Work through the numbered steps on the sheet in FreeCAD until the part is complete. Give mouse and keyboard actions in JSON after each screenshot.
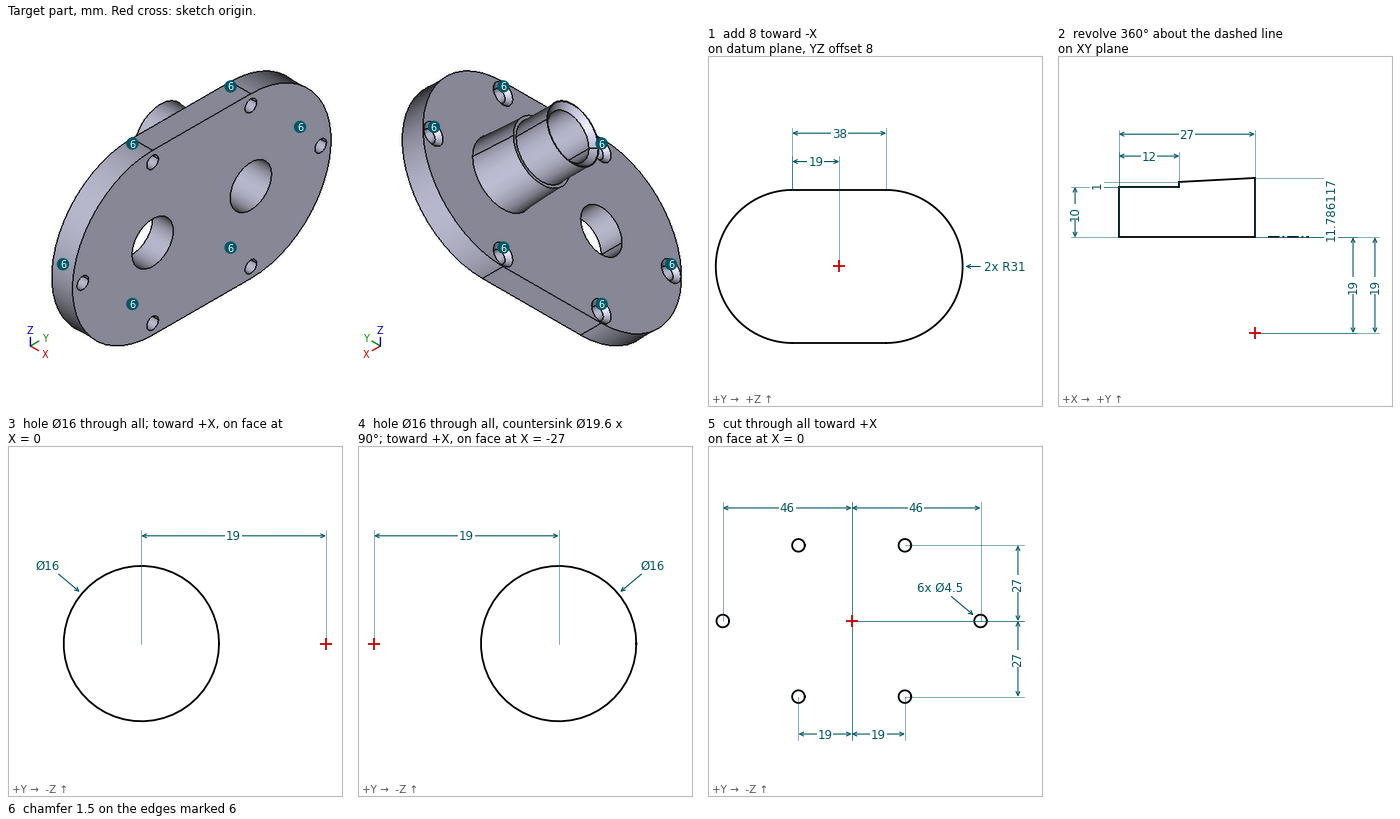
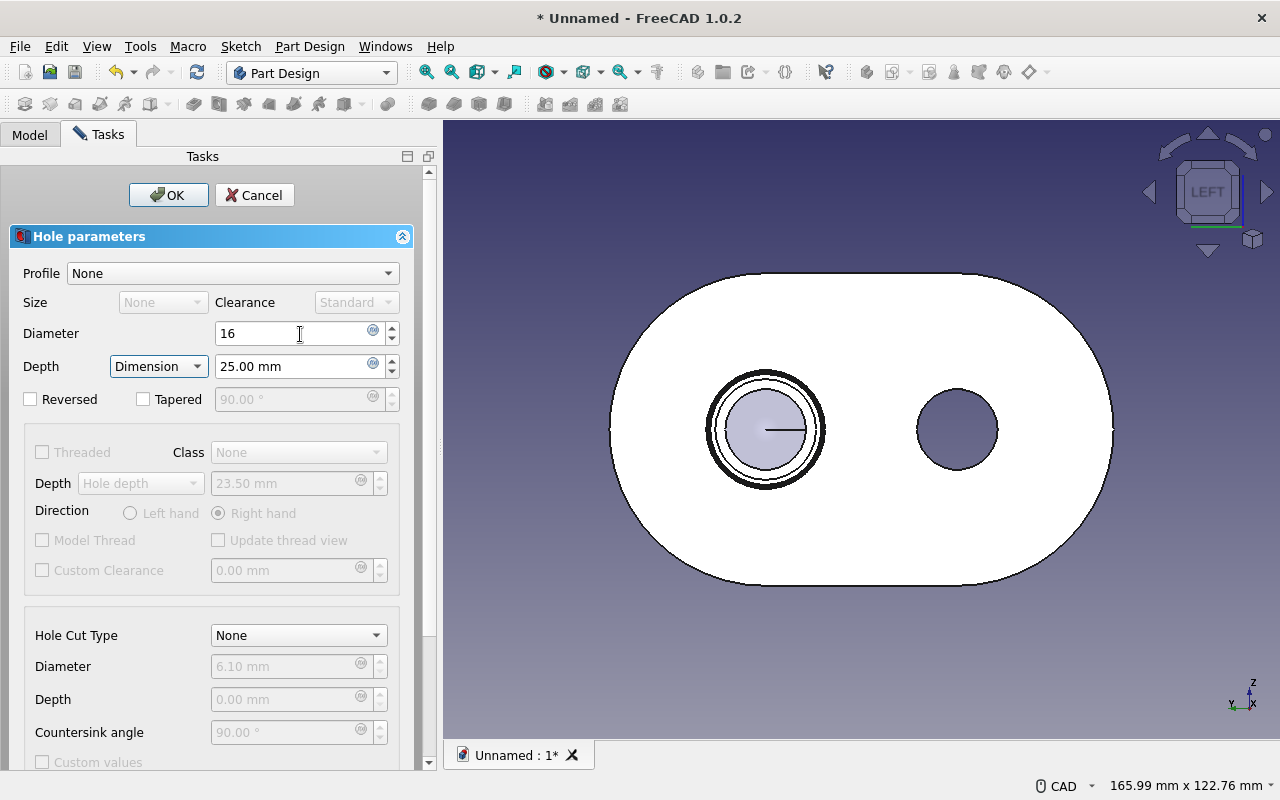
{"action": "left_click", "coordinate": [160, 366]}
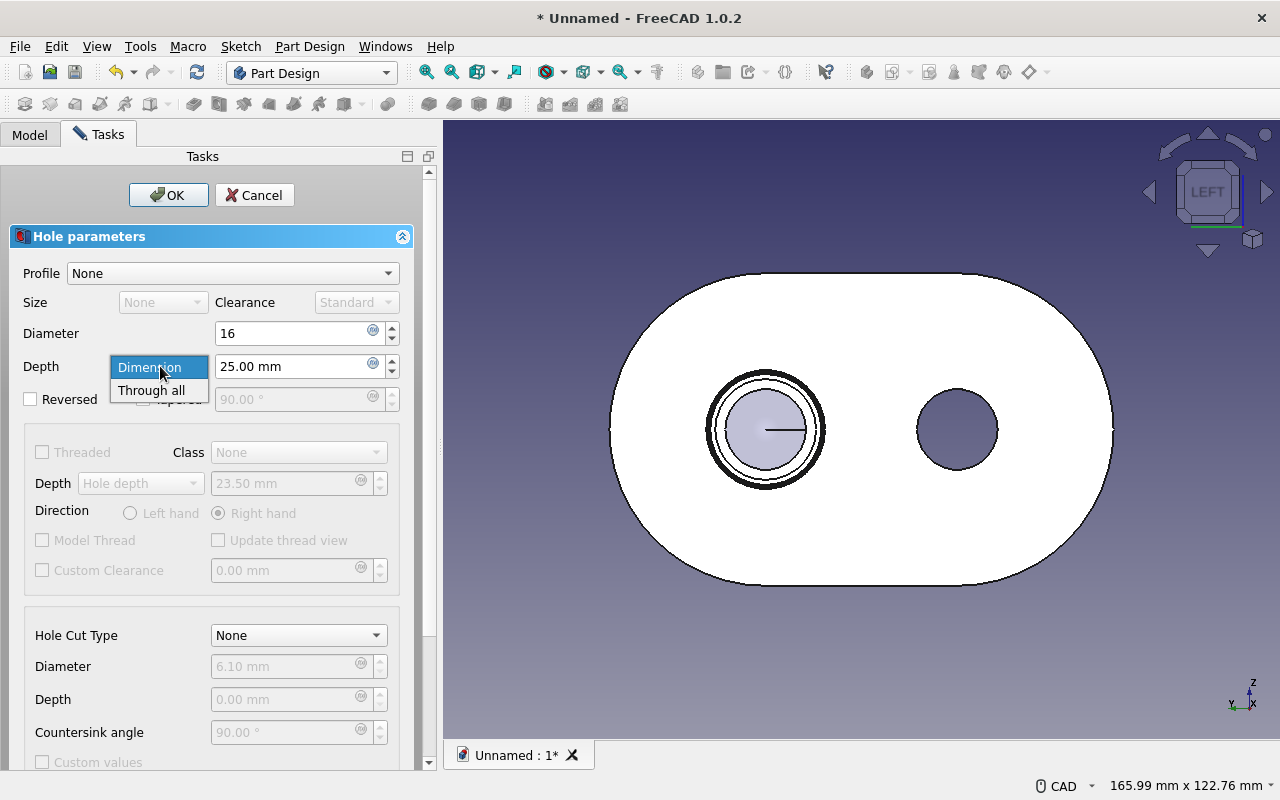
{"action": "left_click", "coordinate": [158, 390]}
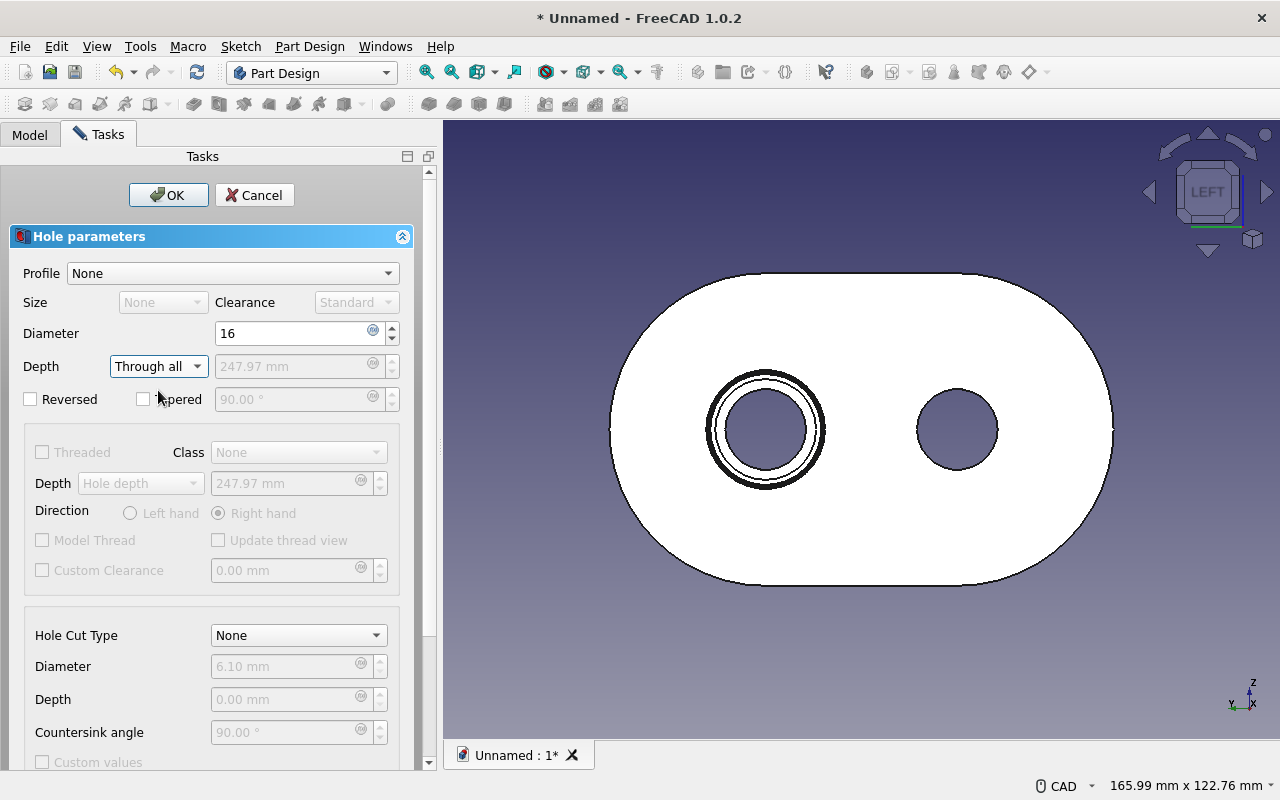
{"action": "left_click", "coordinate": [300, 636]}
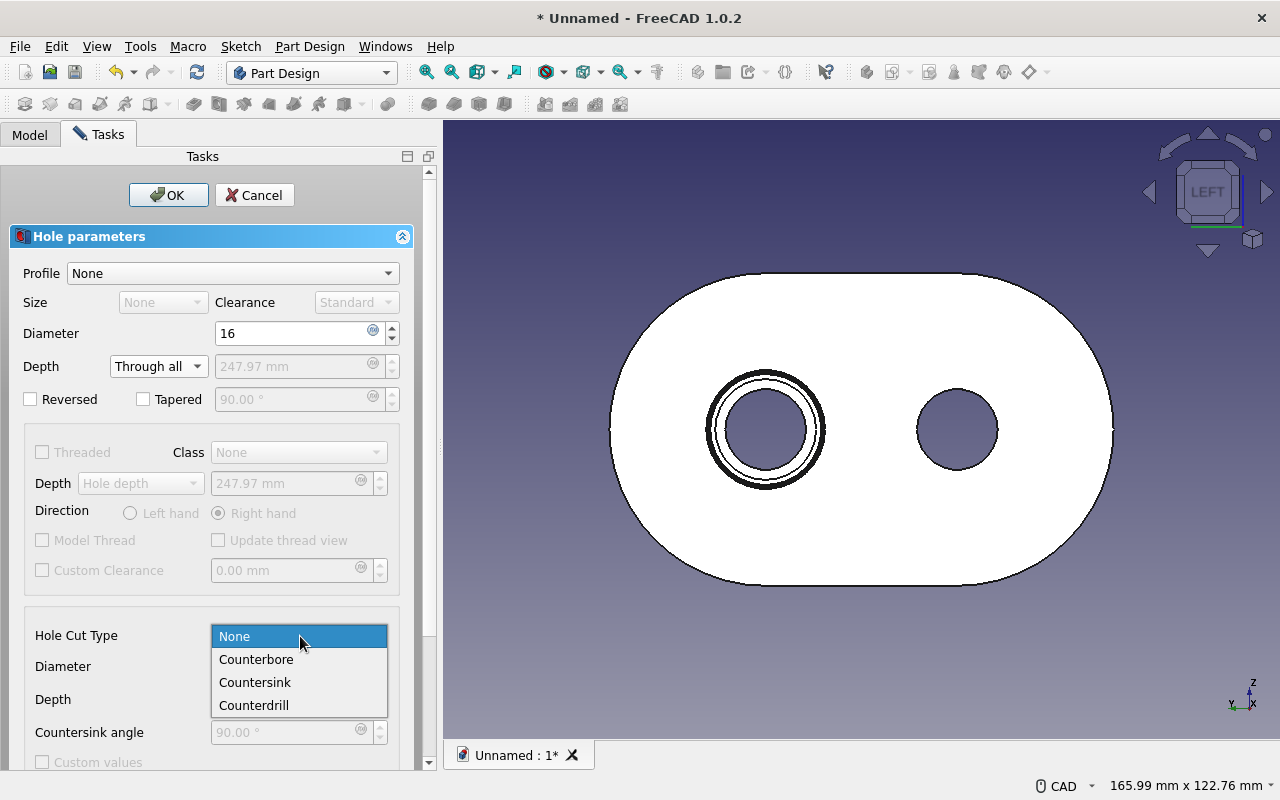
{"action": "left_click", "coordinate": [298, 682]}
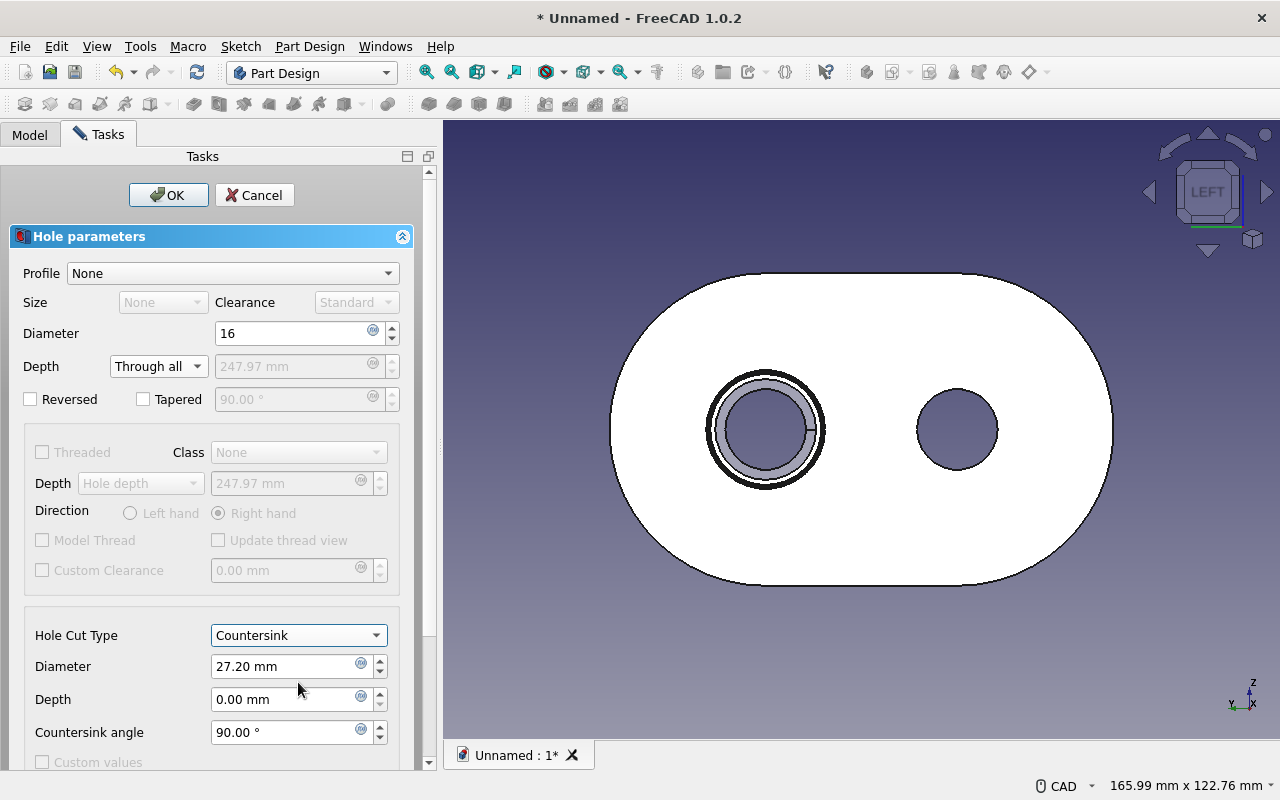
{"action": "triple_click", "coordinate": [292, 666]}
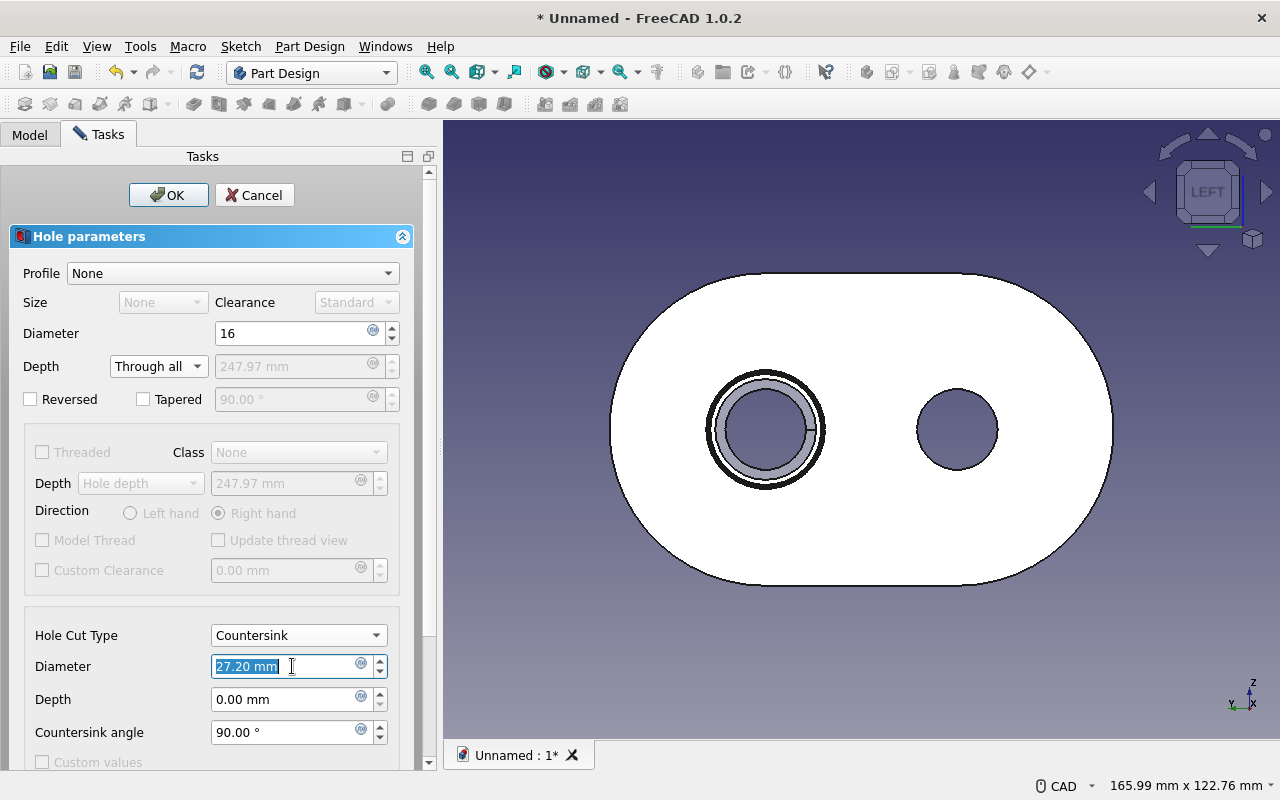
{"action": "type", "text": "19.6"}
{"action": "key", "text": "Tab"}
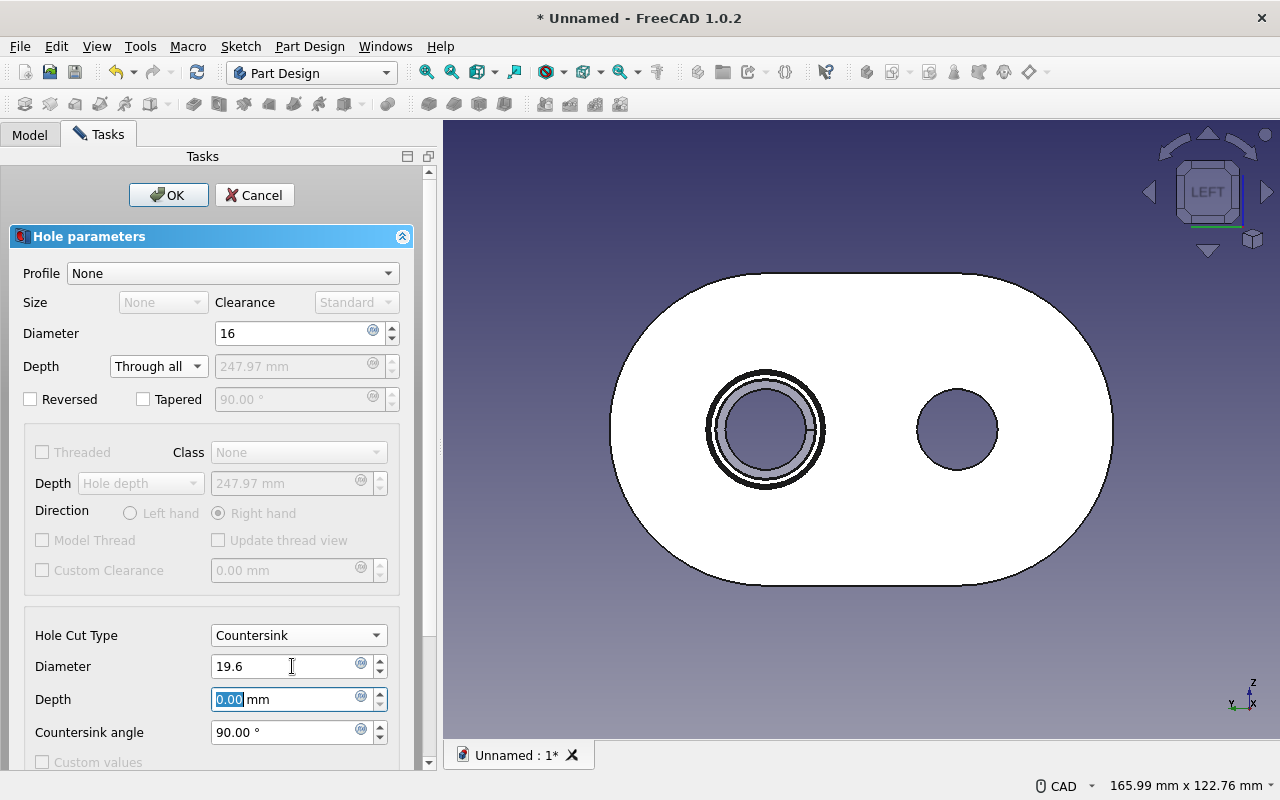
{"action": "left_click", "coordinate": [169, 195]}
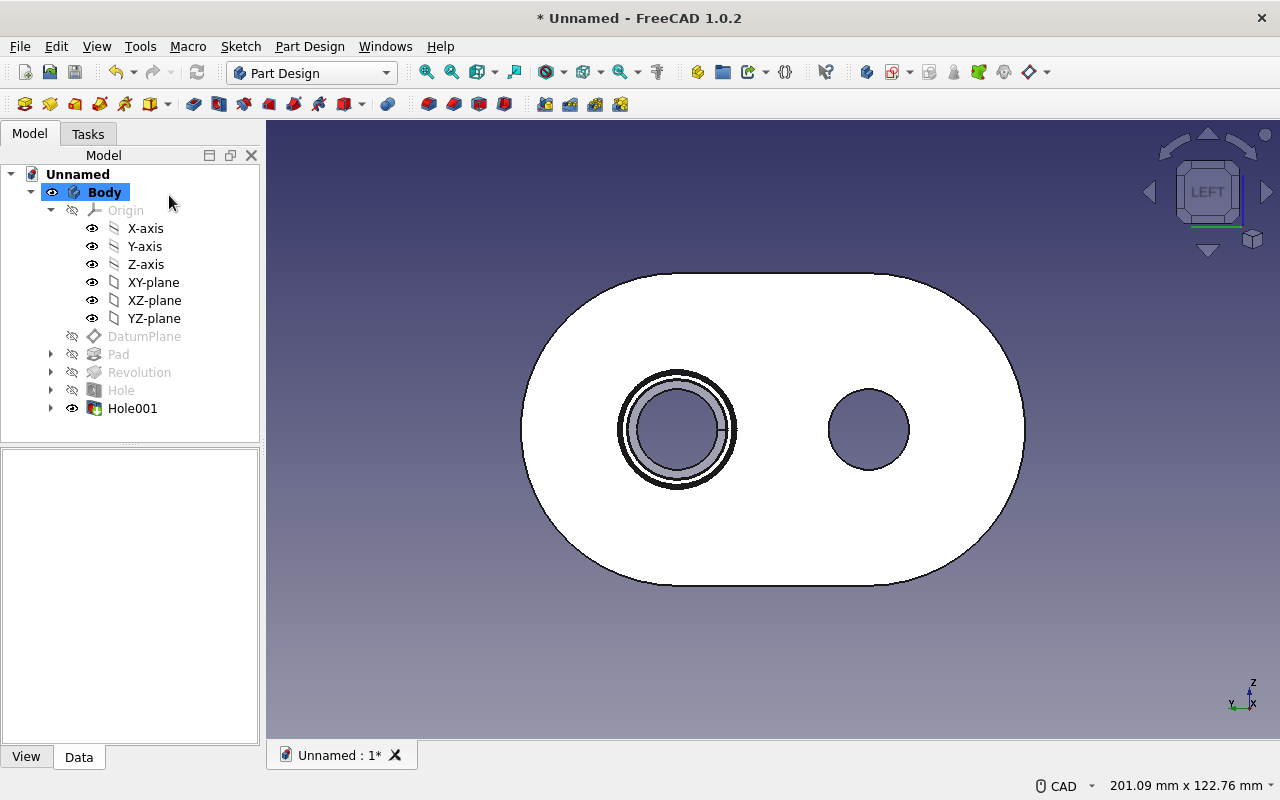
{"action": "left_click", "coordinate": [773, 339]}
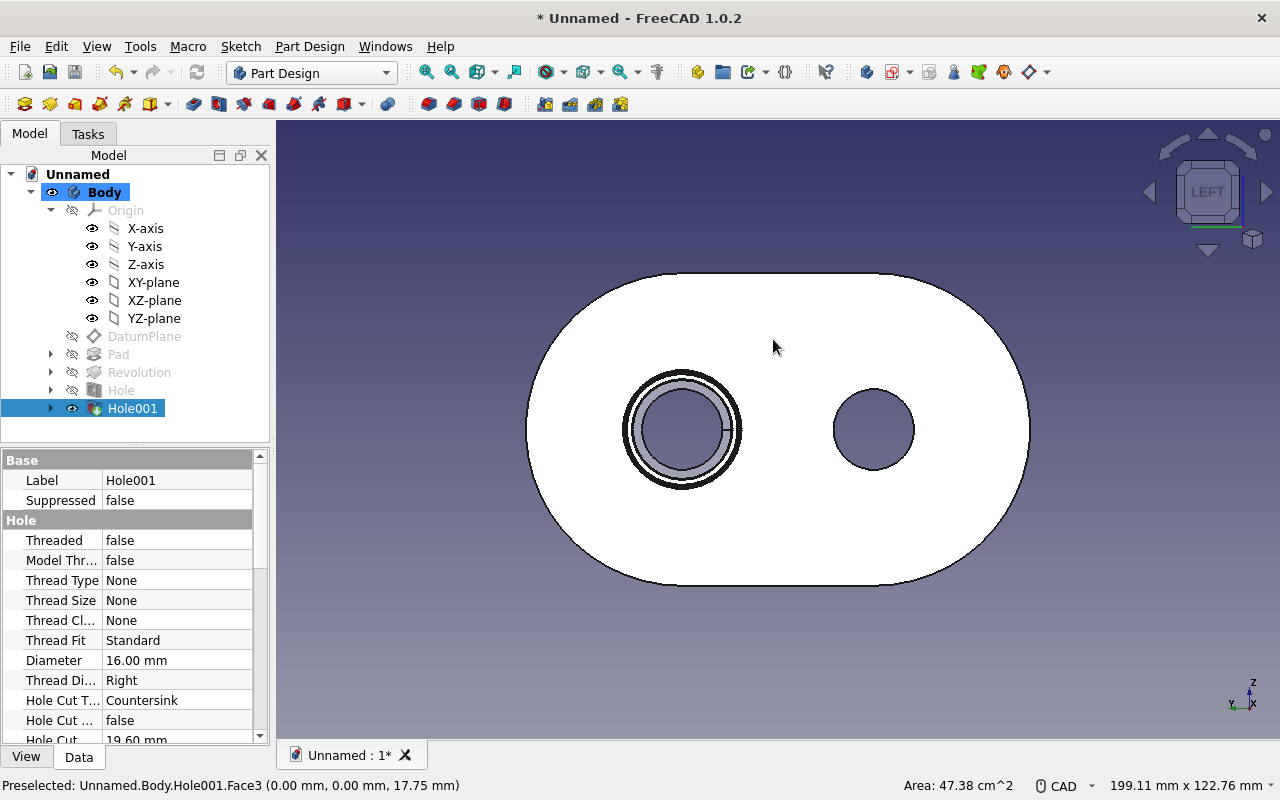
{"action": "left_click", "coordinate": [892, 72]}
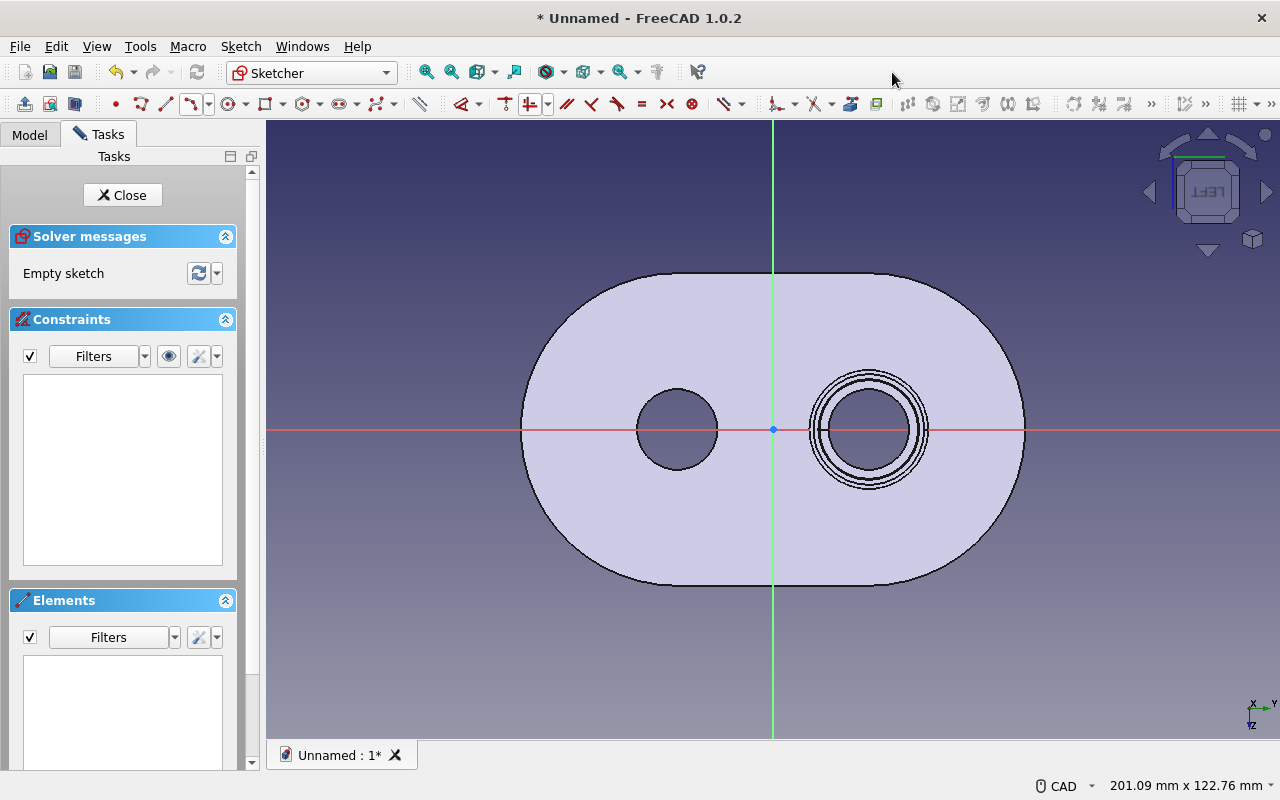
{"action": "left_click", "coordinate": [75, 104]}